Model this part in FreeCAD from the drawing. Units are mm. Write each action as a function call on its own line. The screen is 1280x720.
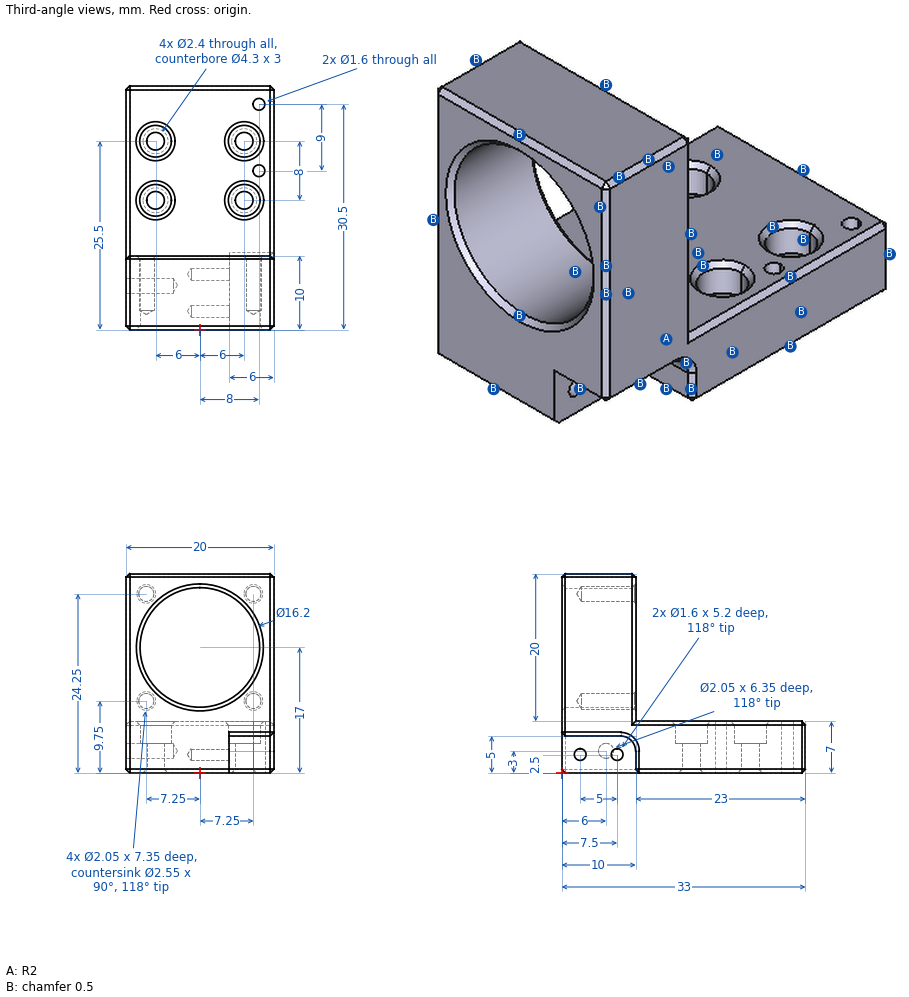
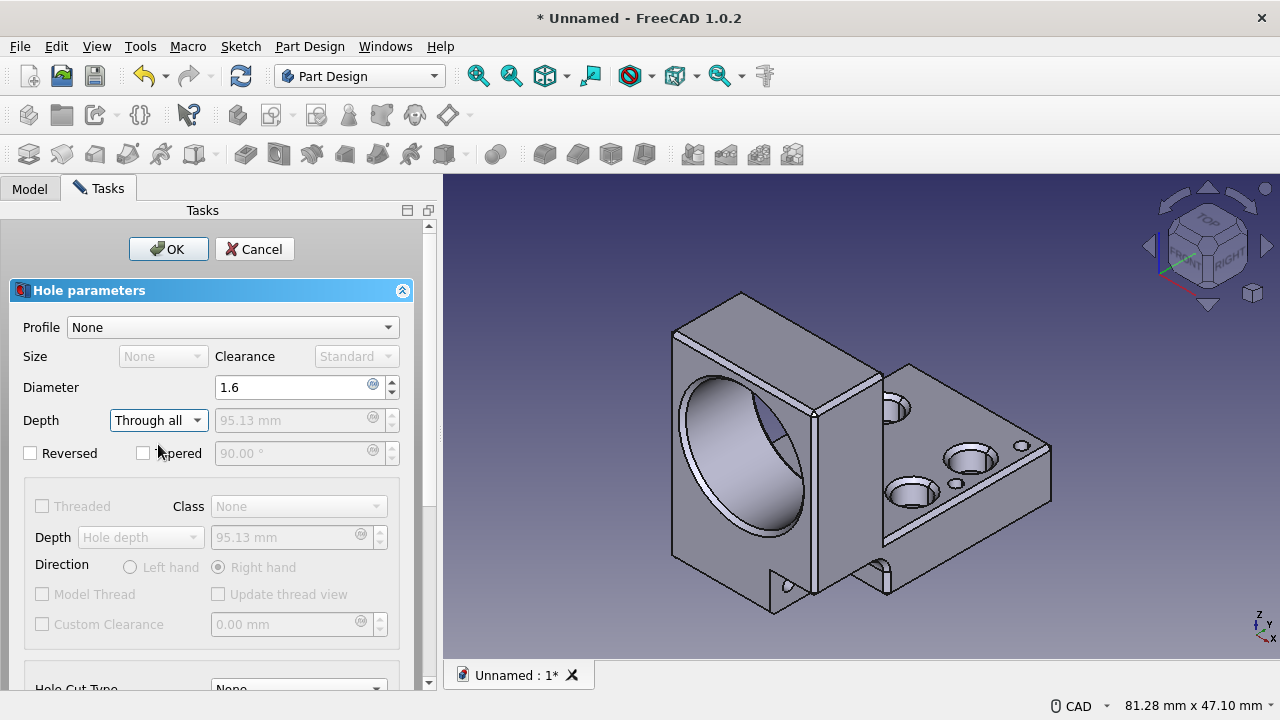
click(169, 249)